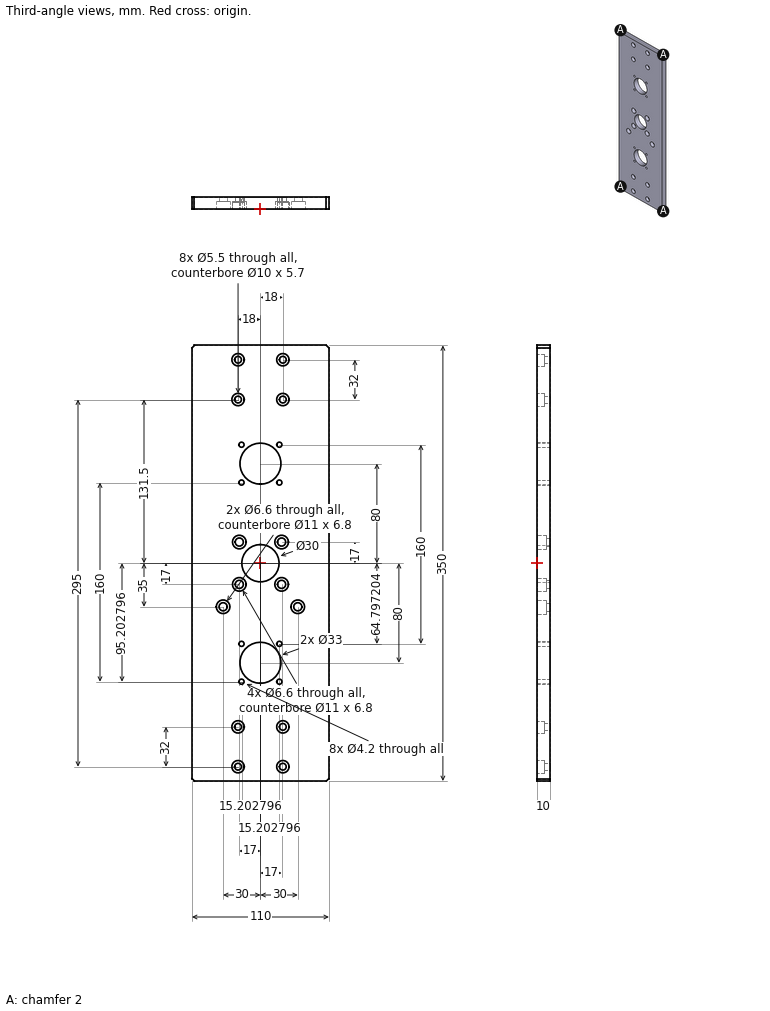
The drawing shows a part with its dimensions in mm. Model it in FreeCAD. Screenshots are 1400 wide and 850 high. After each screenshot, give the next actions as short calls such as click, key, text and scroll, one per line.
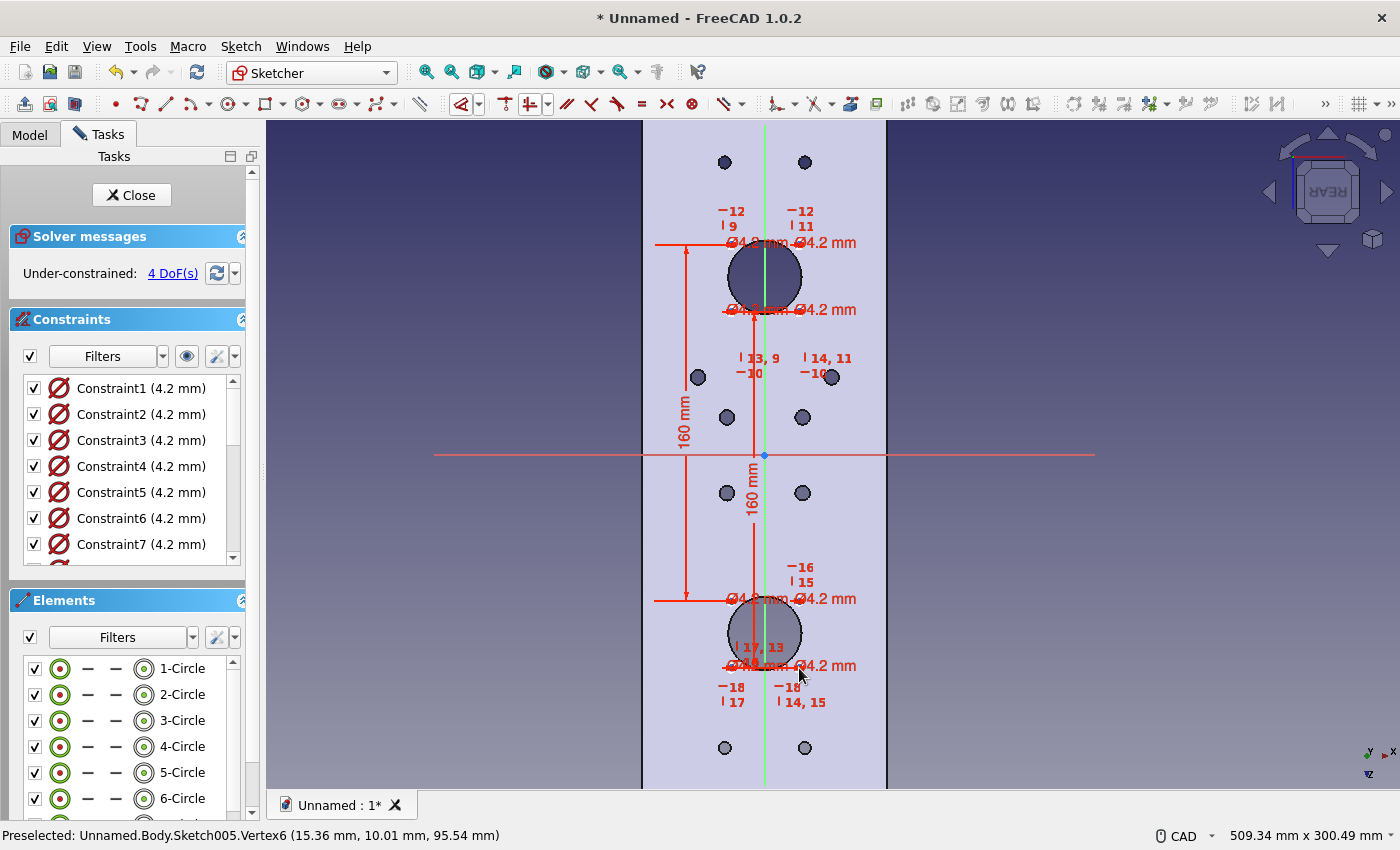
click(731, 245)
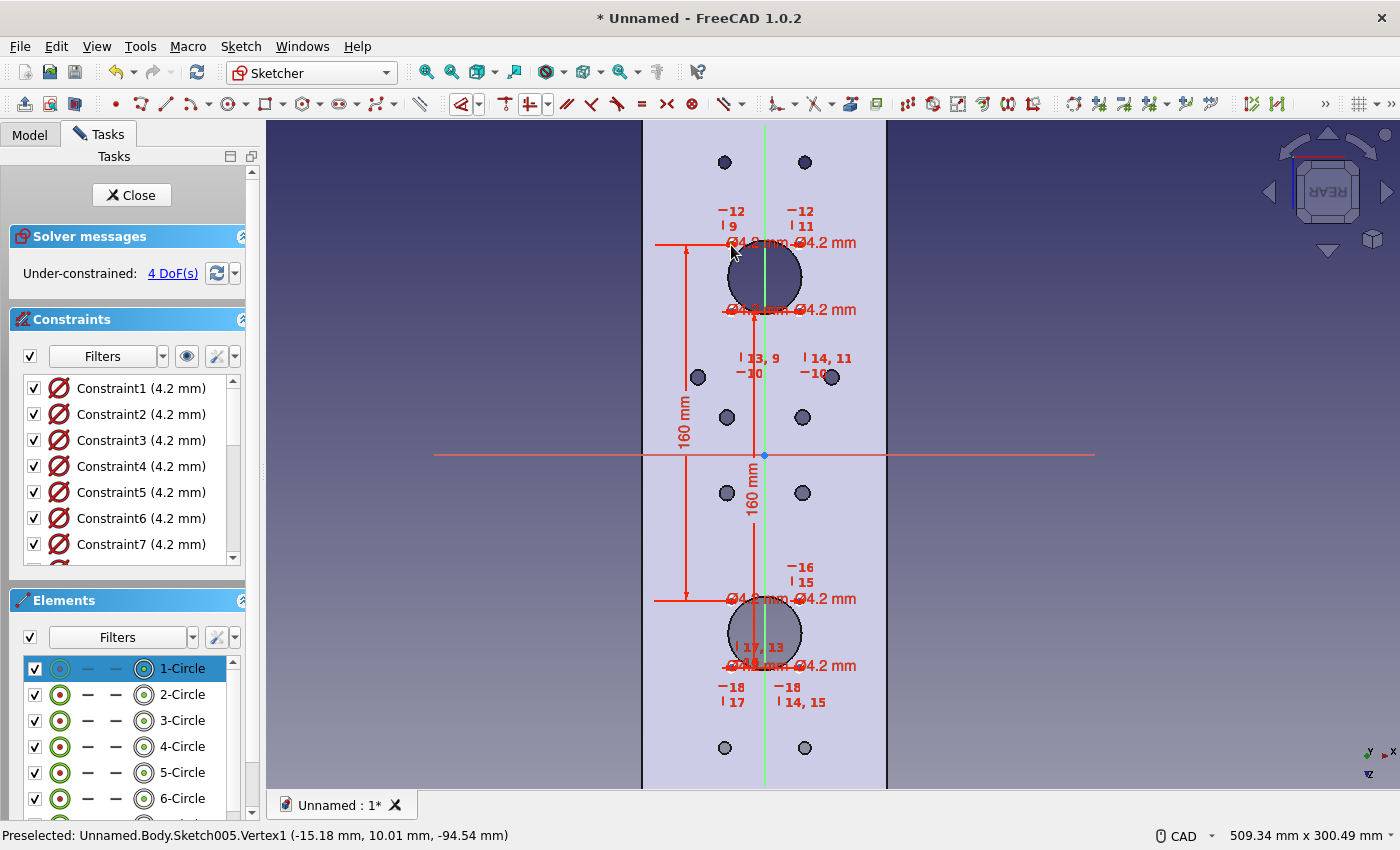
key(l)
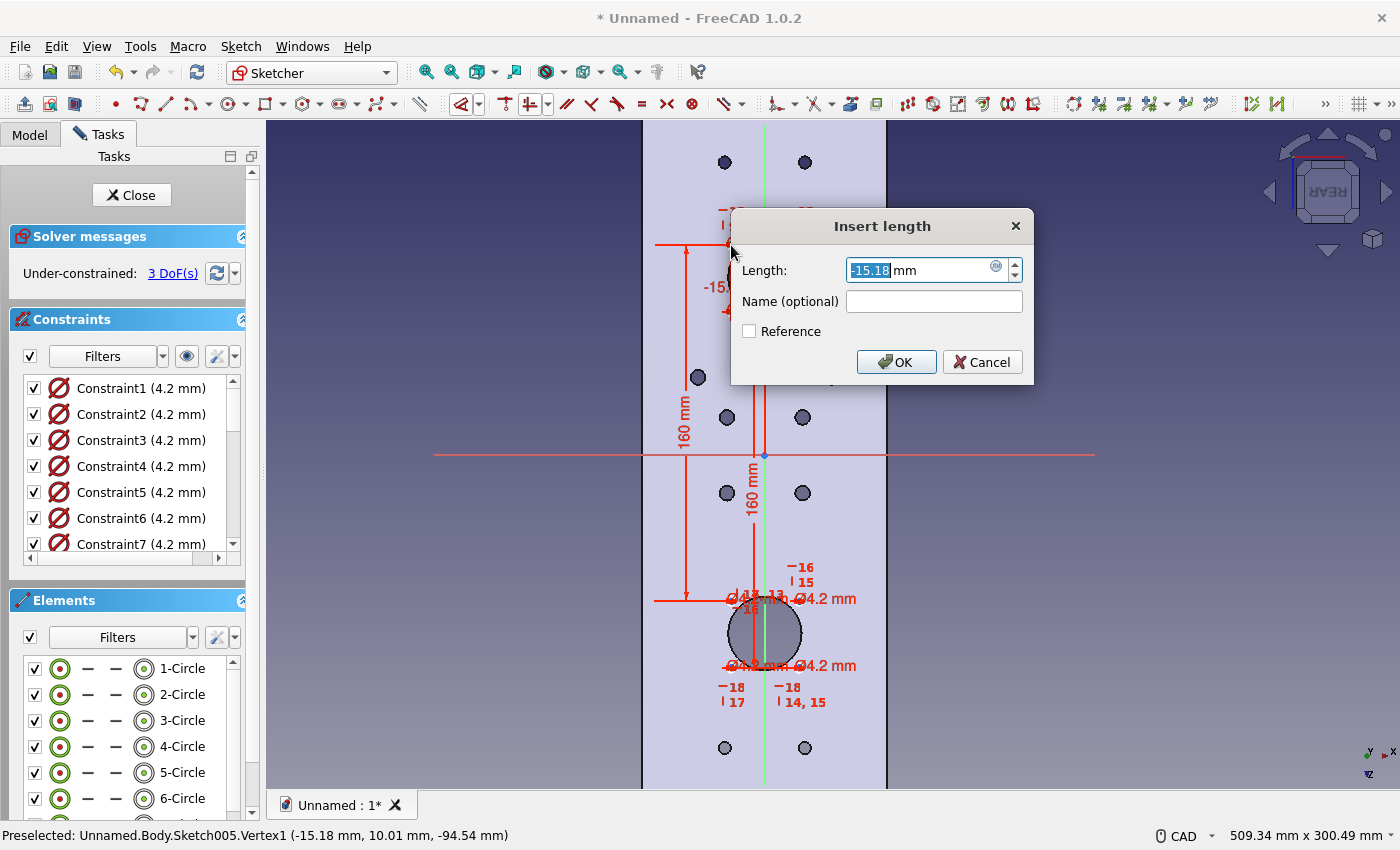
text(-15.202796)
key(Return)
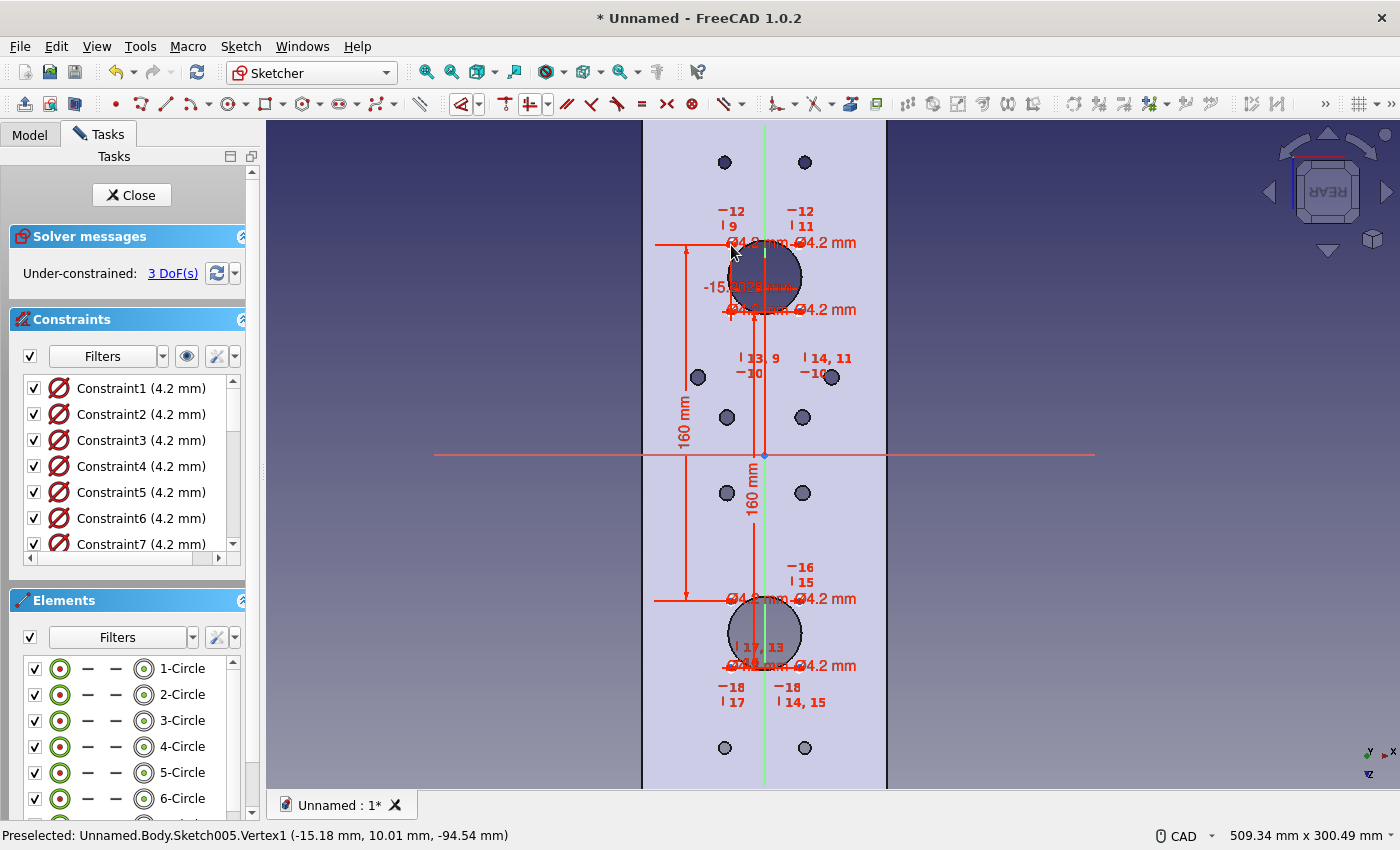
click(731, 245)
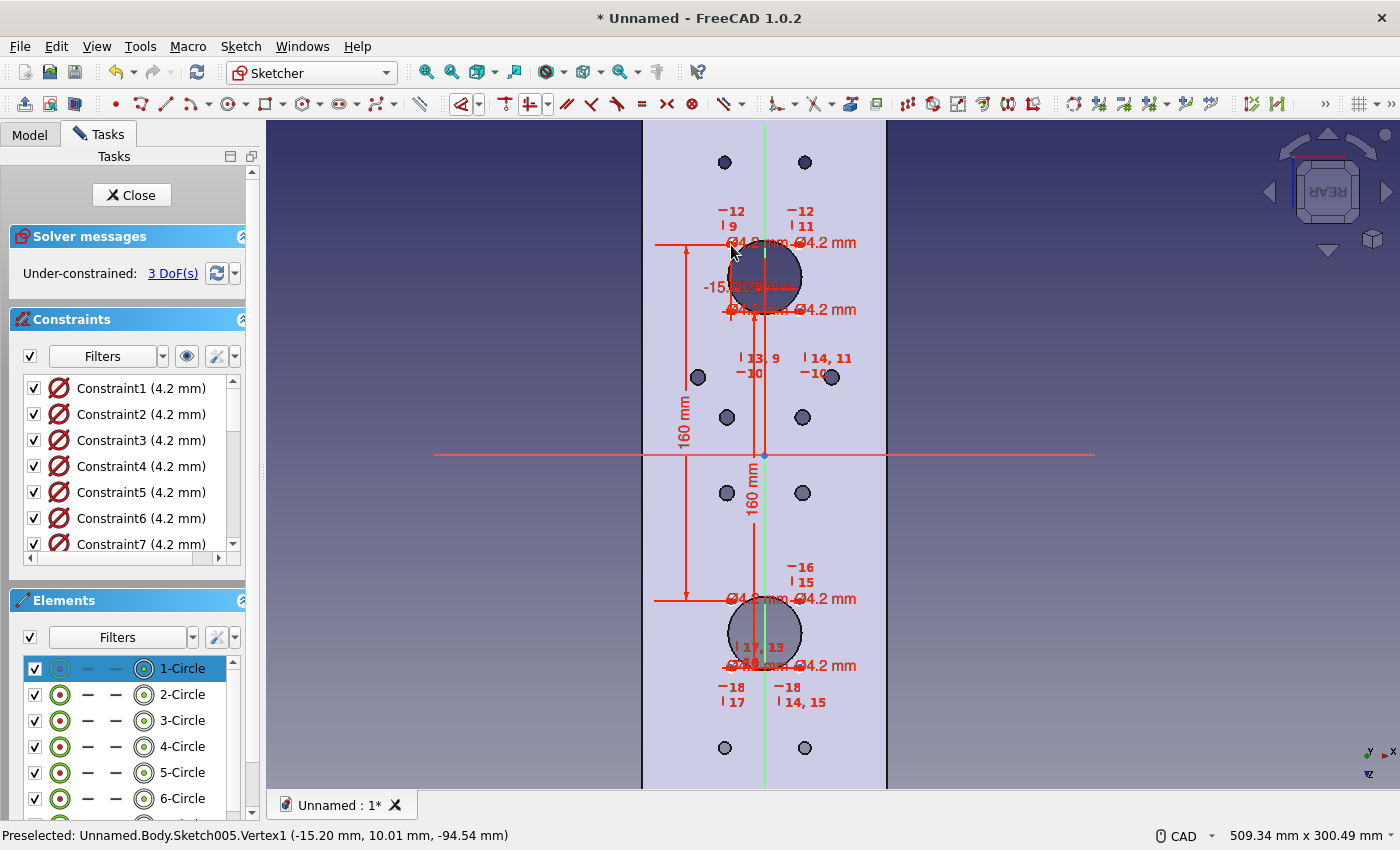
key(i)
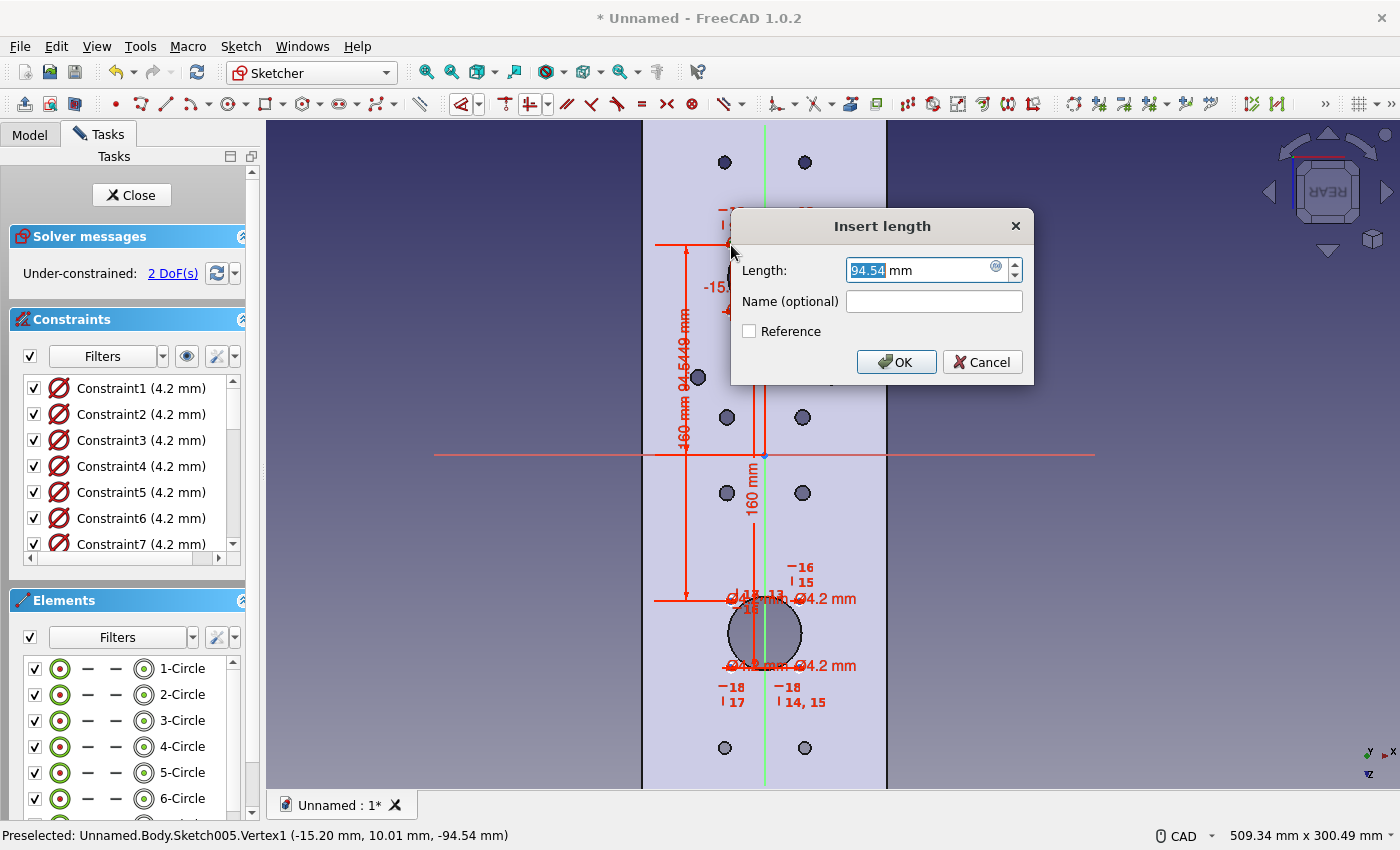
text(95.202796)
key(Return)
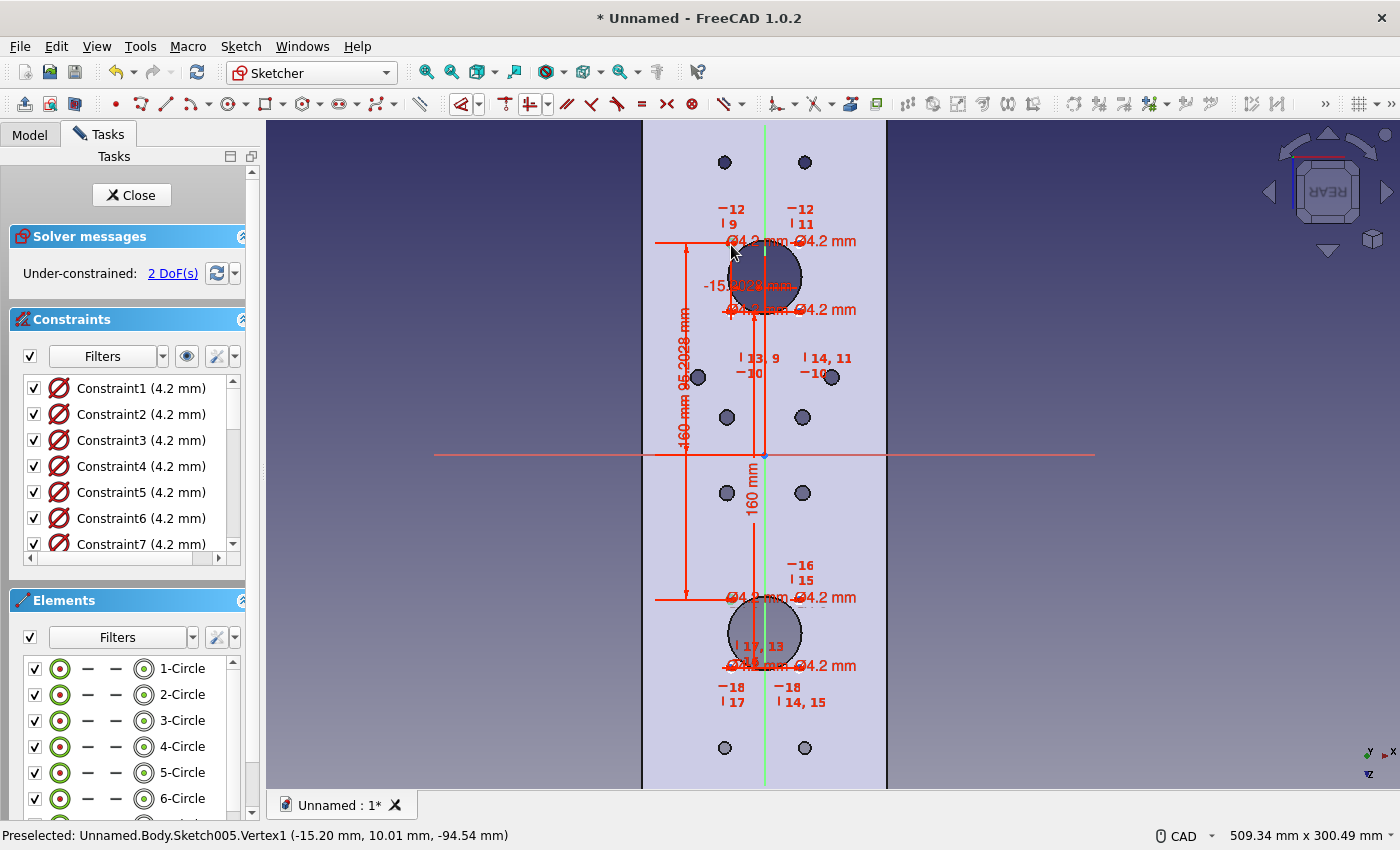
click(799, 312)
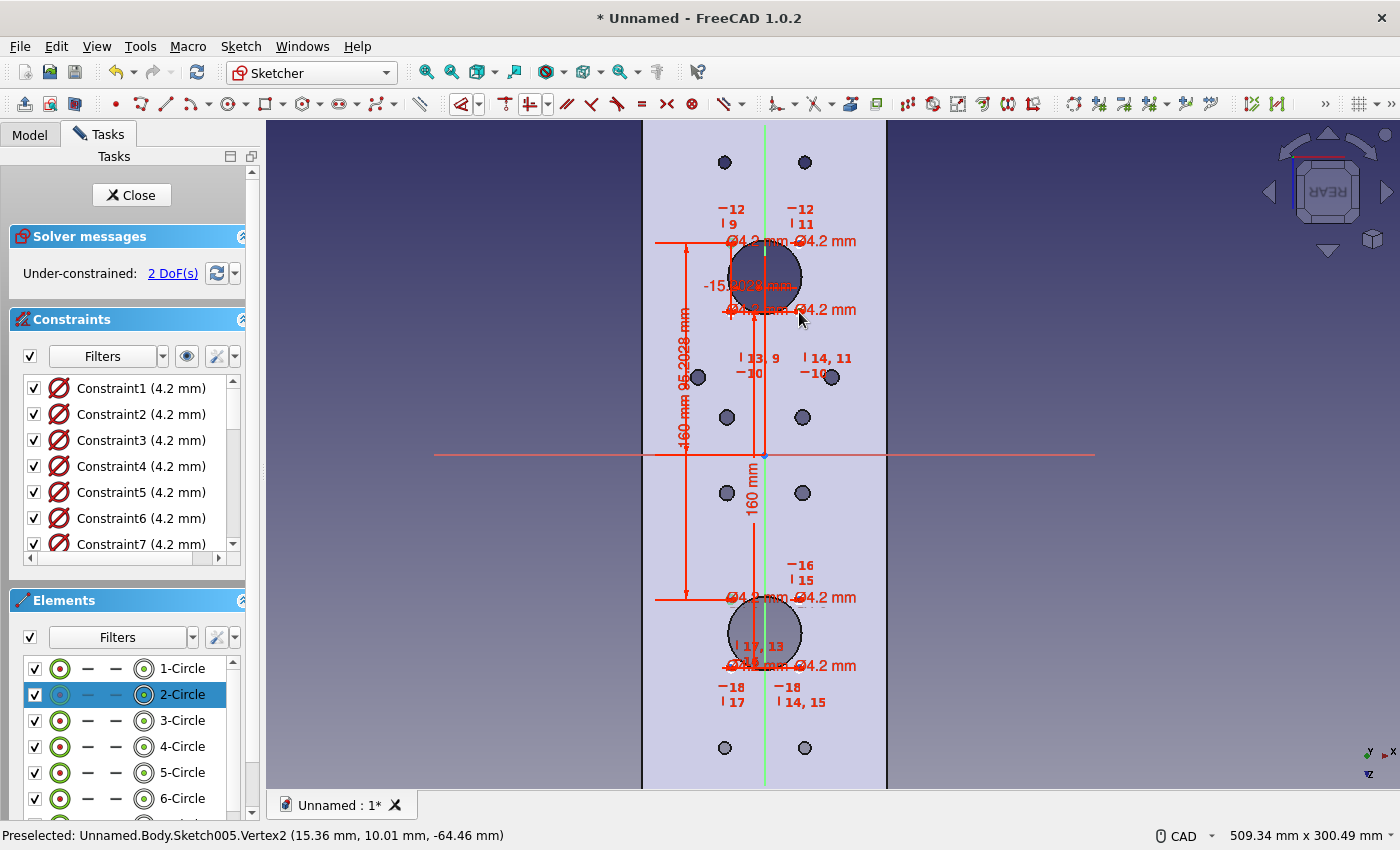
key(l)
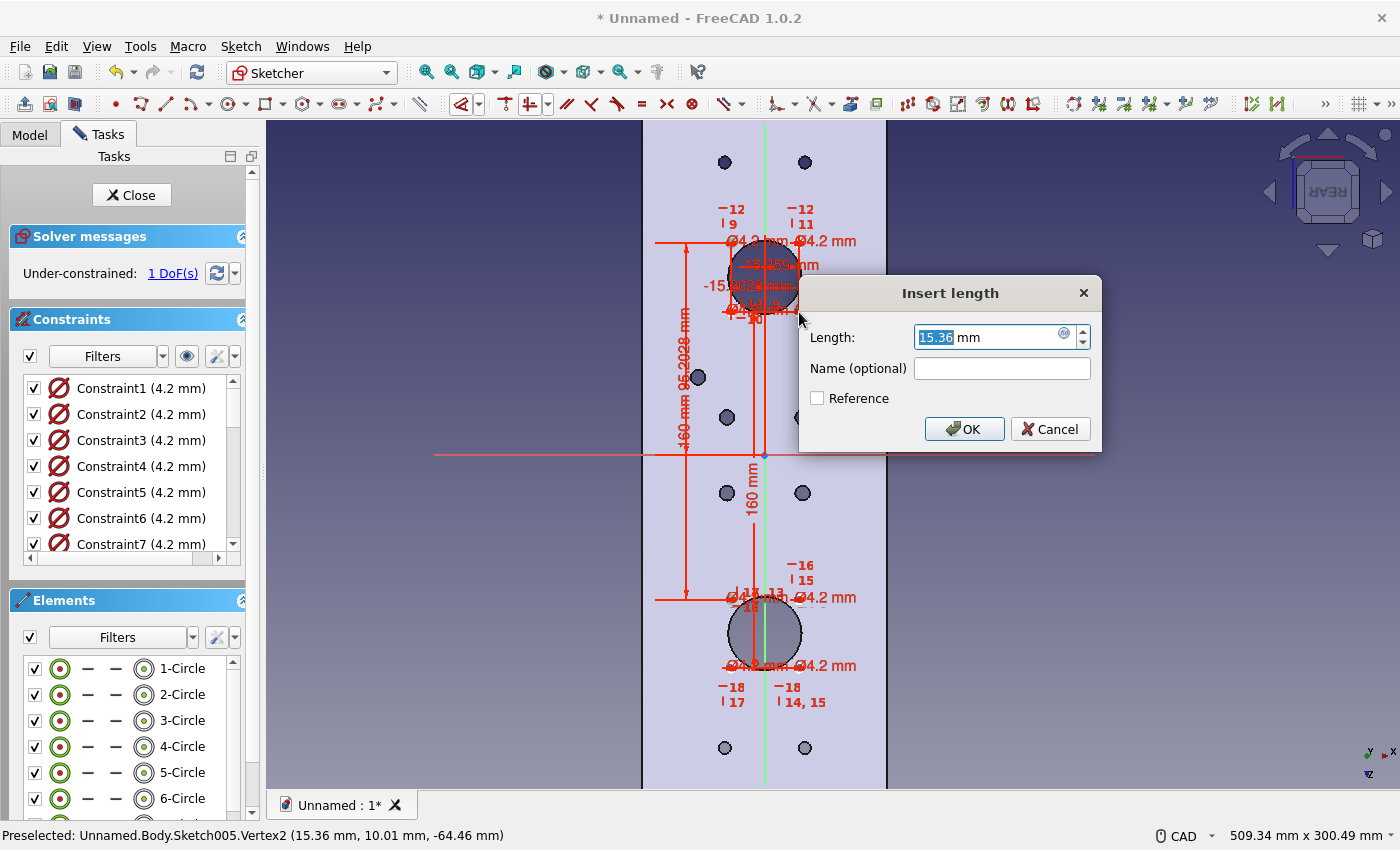
text(15.202796)
key(Return)